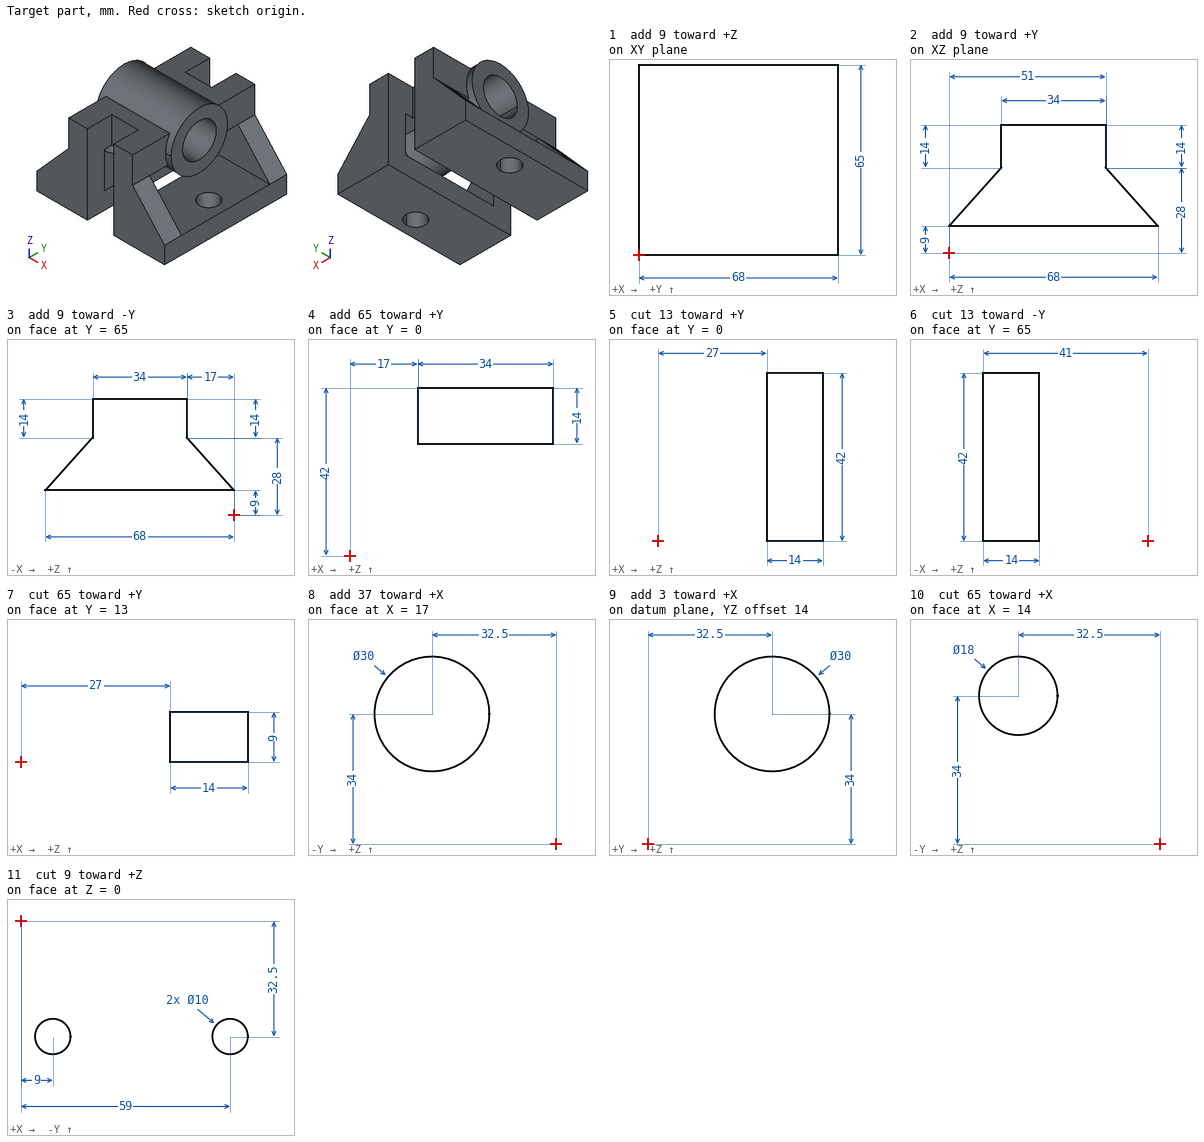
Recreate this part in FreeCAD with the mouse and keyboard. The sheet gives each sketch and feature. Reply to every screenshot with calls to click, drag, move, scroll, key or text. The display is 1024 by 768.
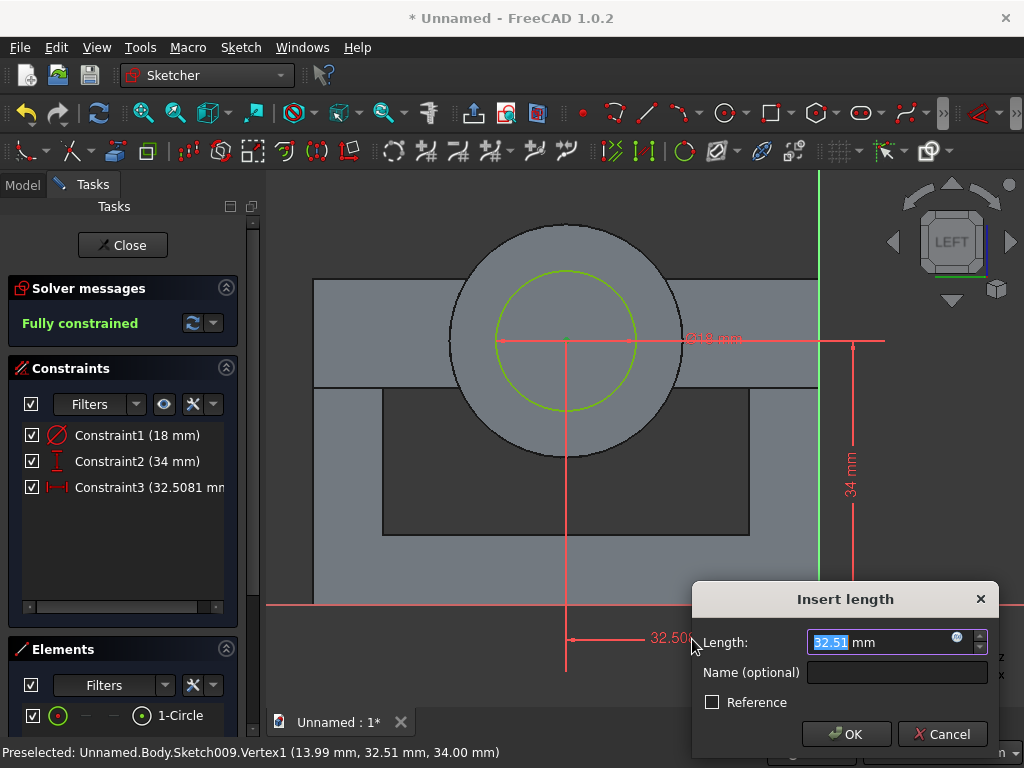
text(32.5)
key(Return)
key(Escape)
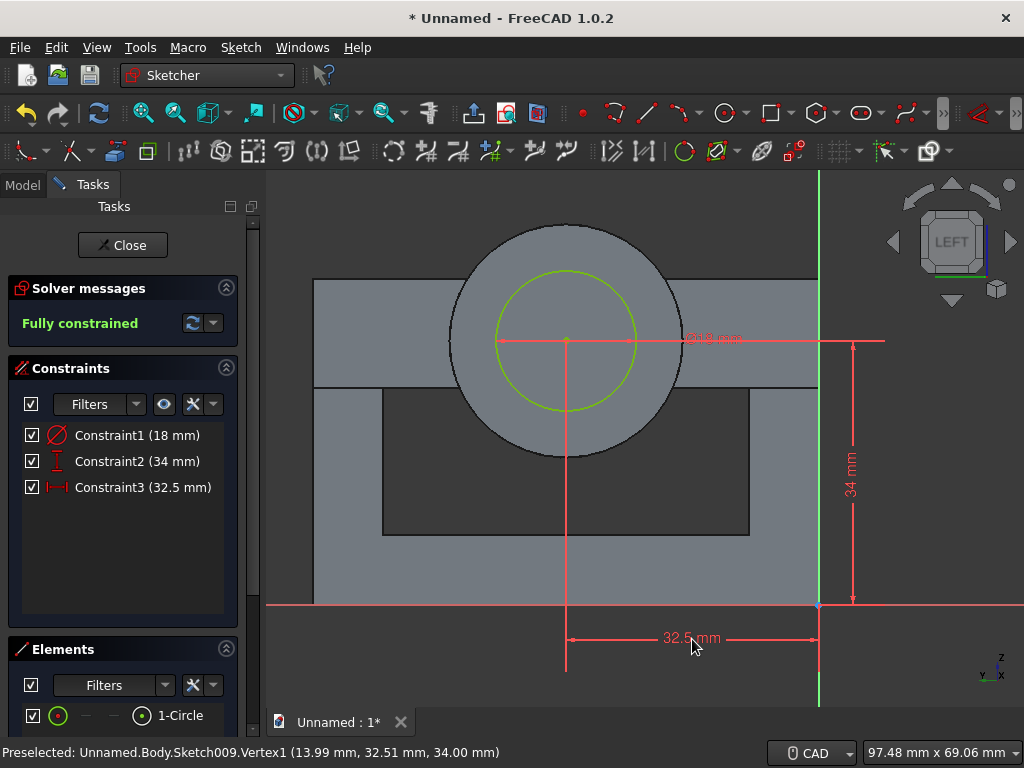
click(123, 245)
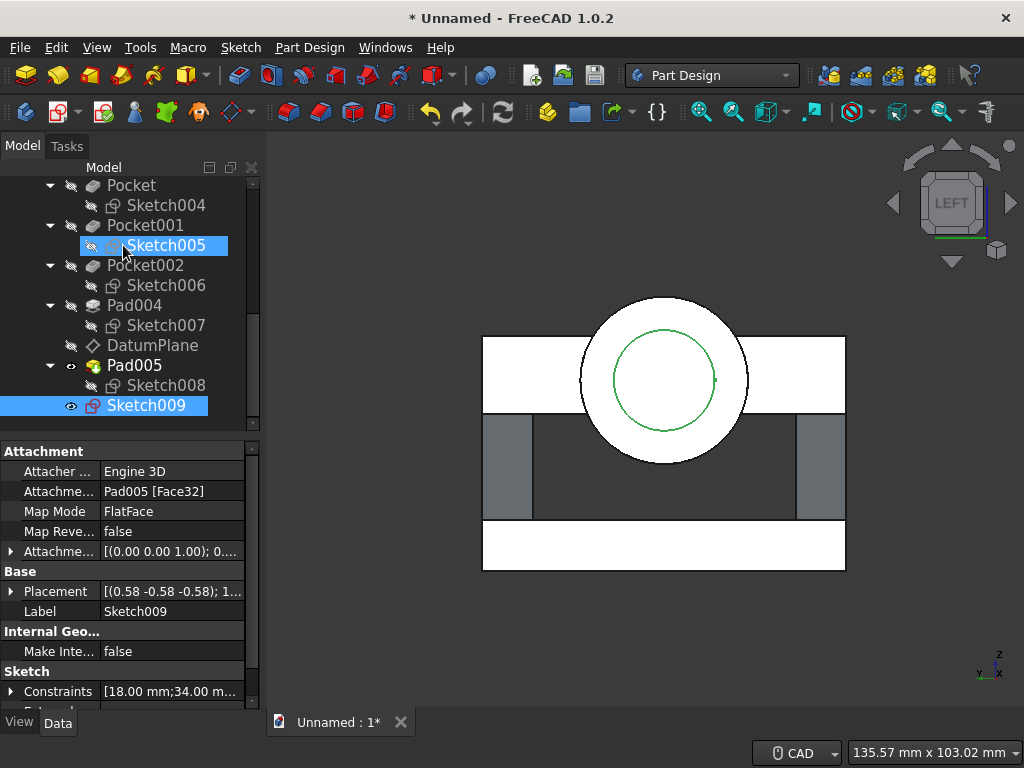
click(240, 76)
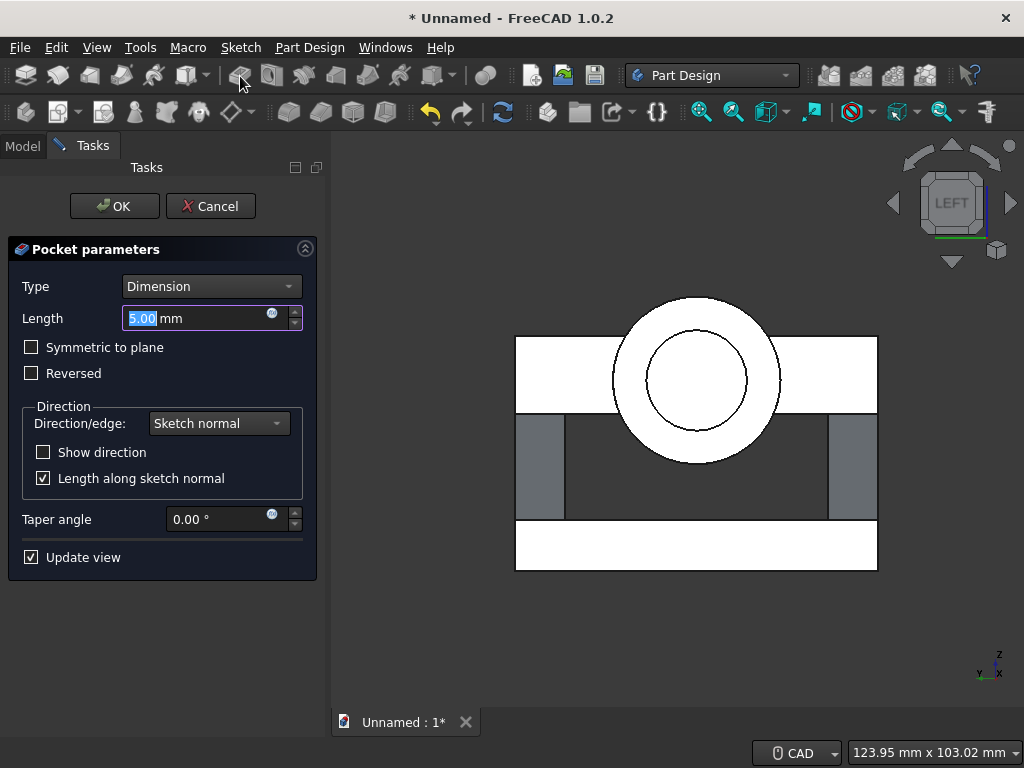
text(65)
key(Tab)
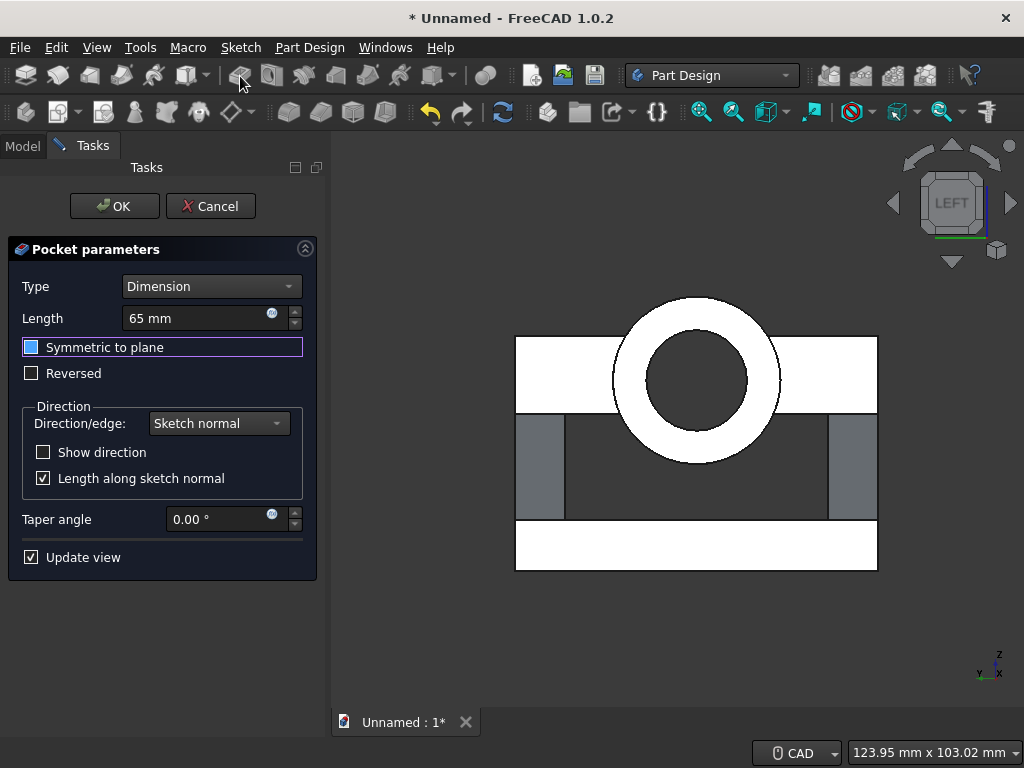
click(115, 206)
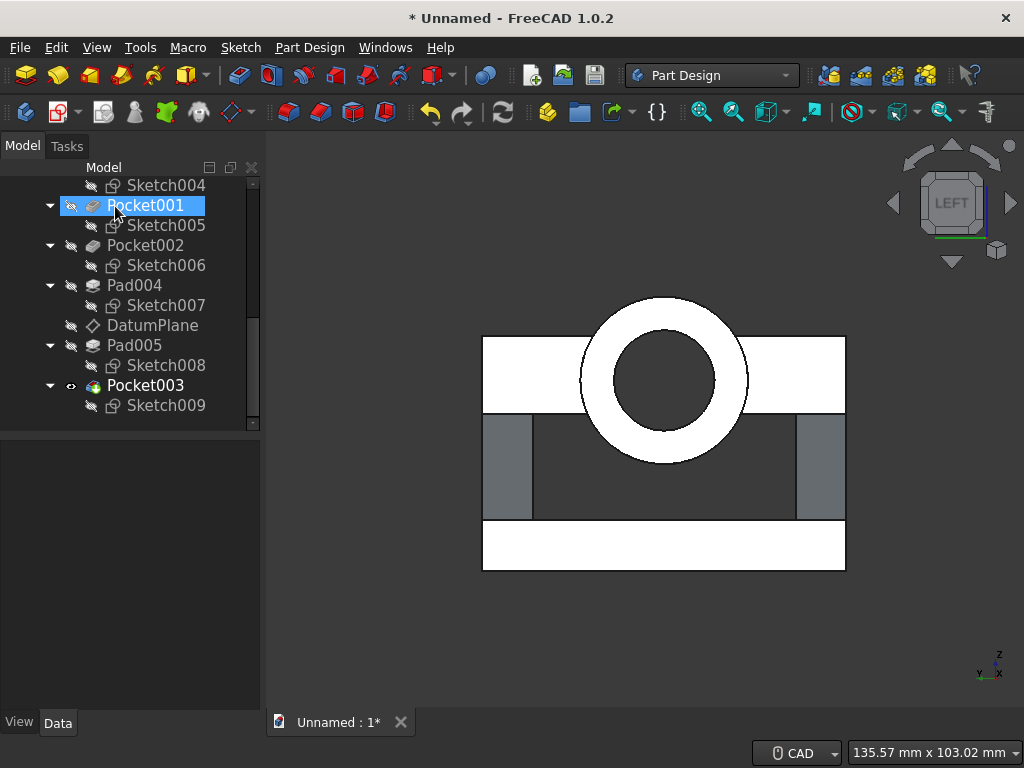
key(5)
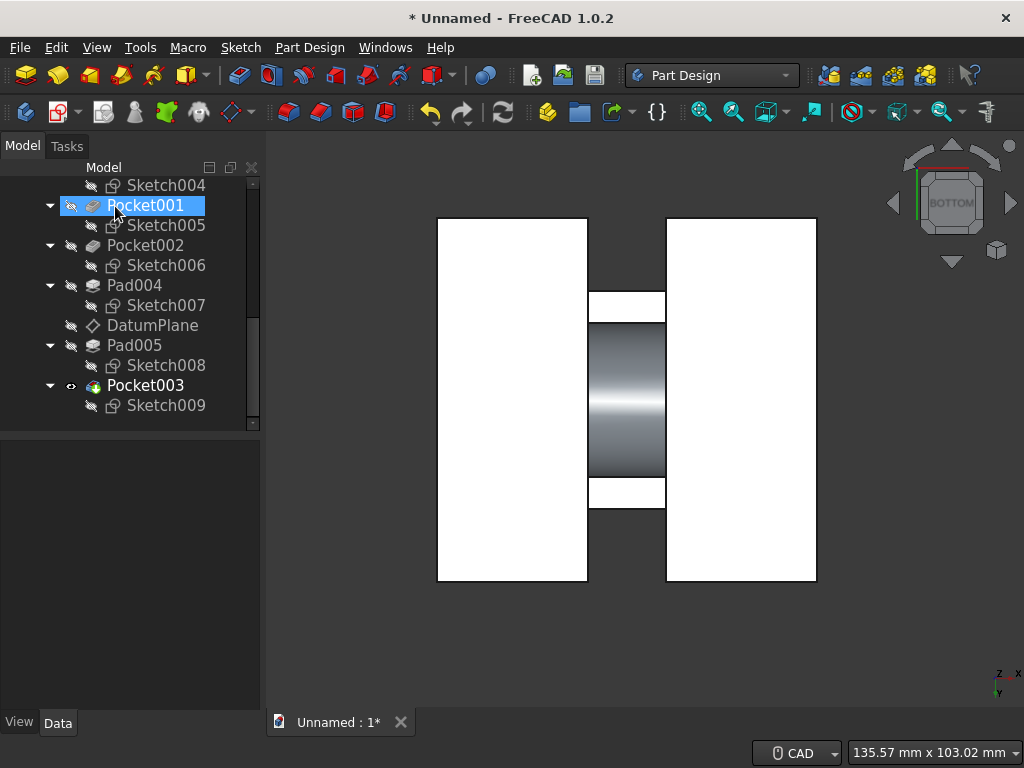
click(742, 503)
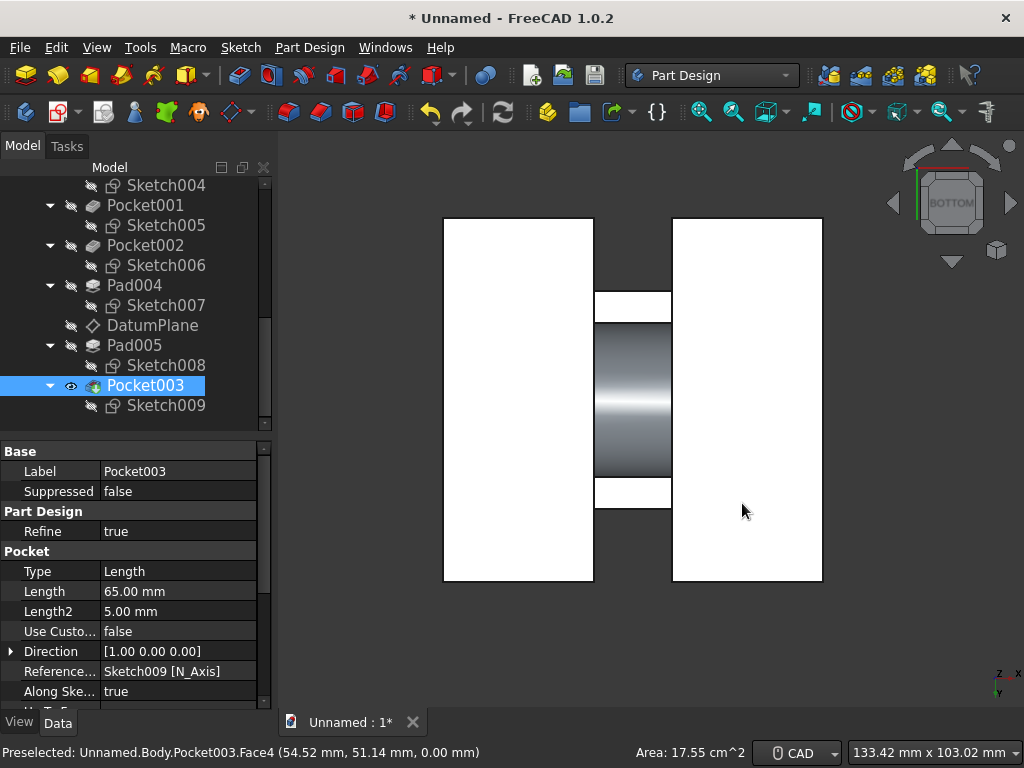
click(58, 112)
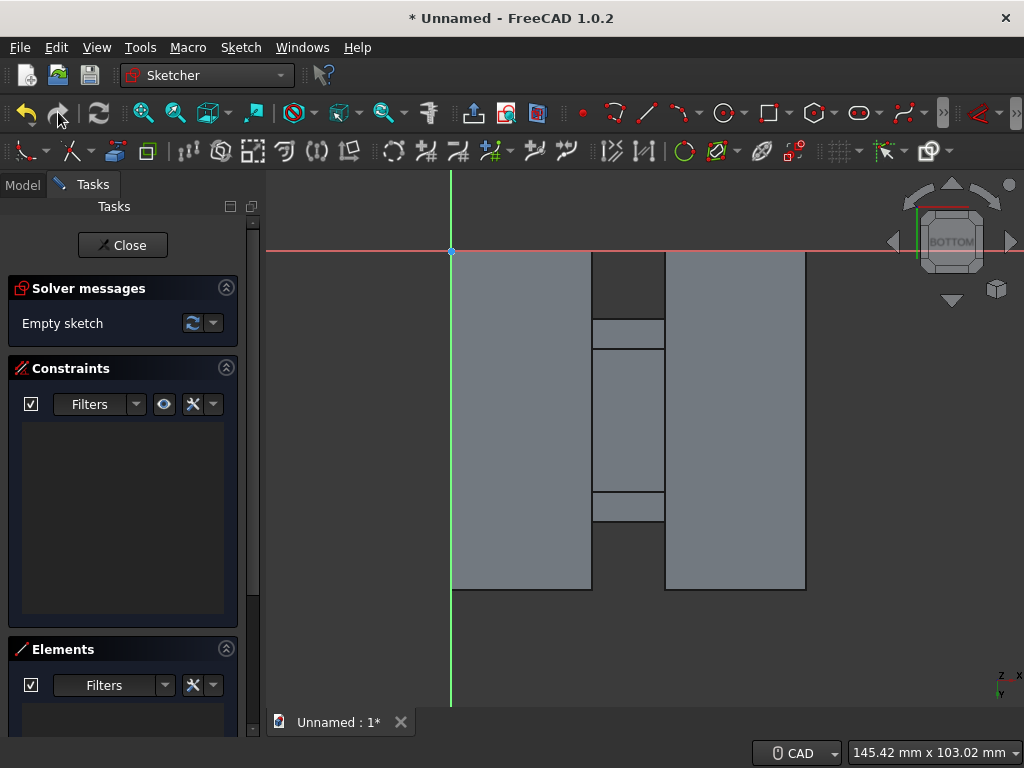
click(724, 114)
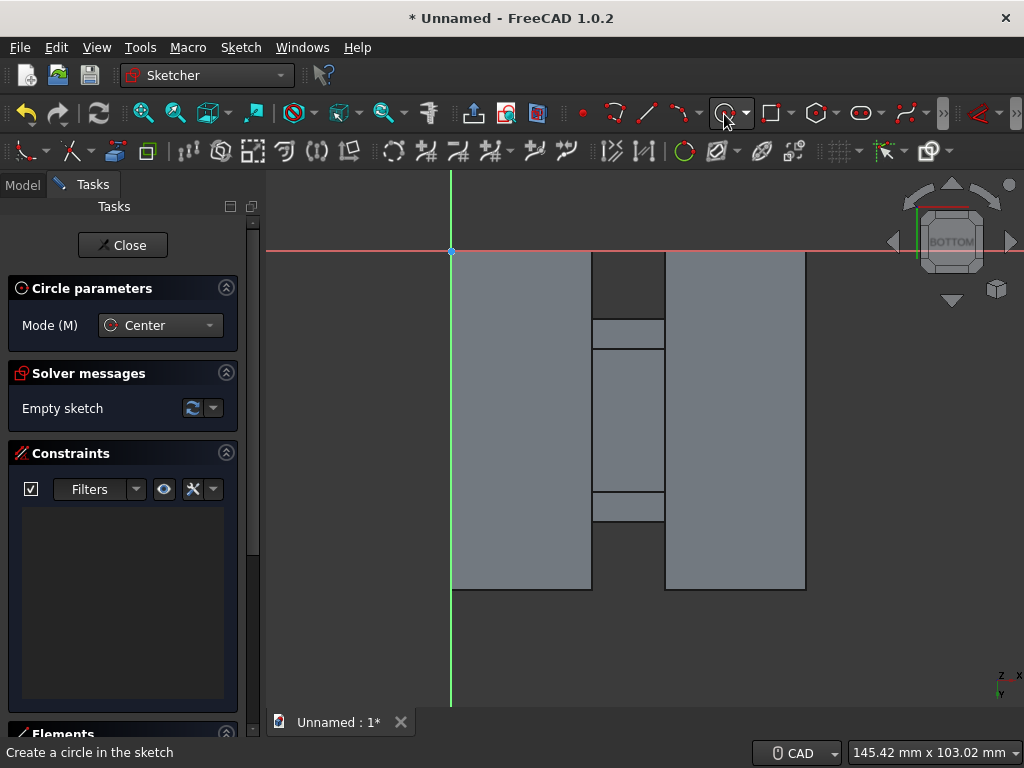
click(759, 421)
move(777, 402)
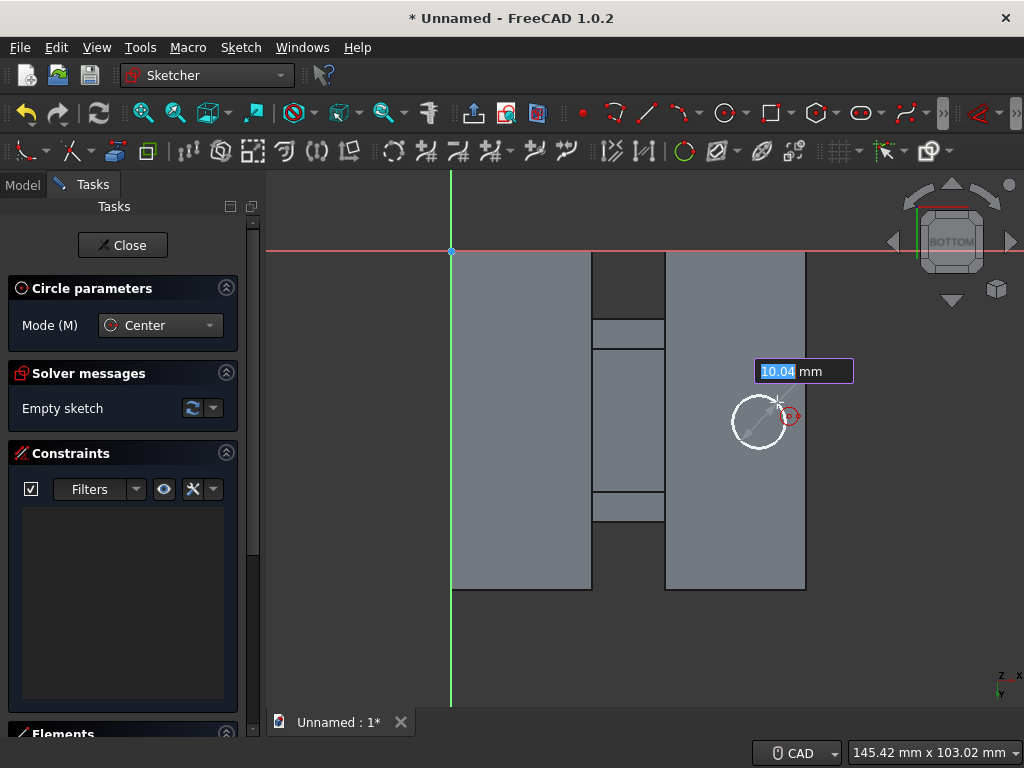
text(10)
key(Return)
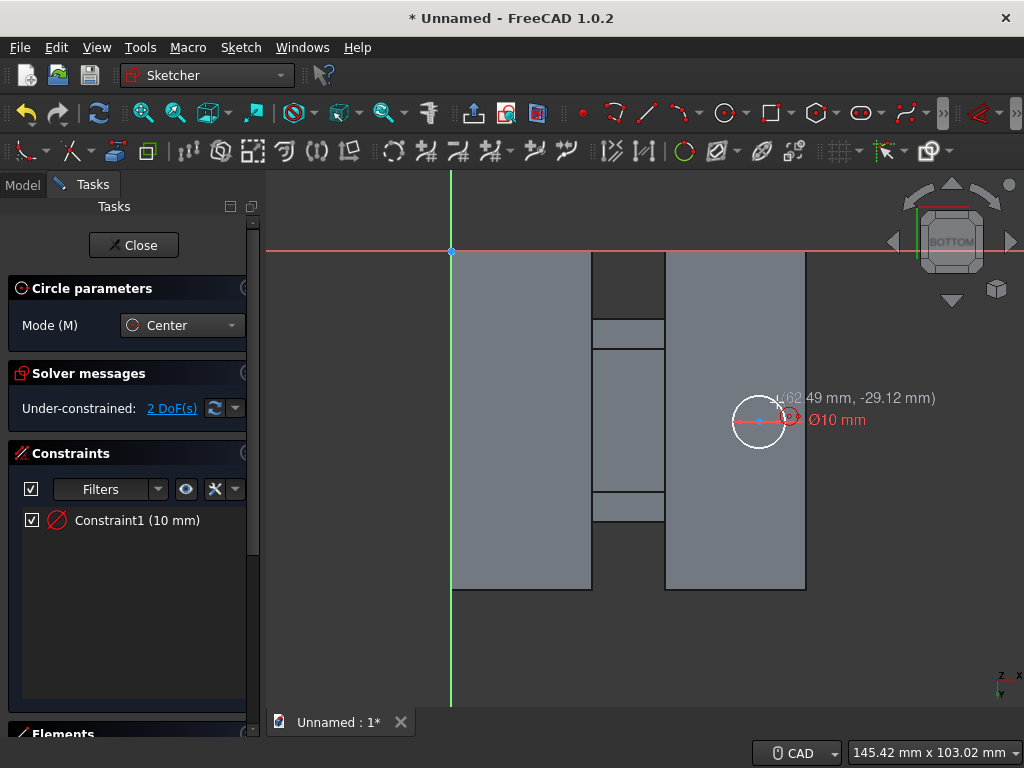
click(498, 421)
move(517, 402)